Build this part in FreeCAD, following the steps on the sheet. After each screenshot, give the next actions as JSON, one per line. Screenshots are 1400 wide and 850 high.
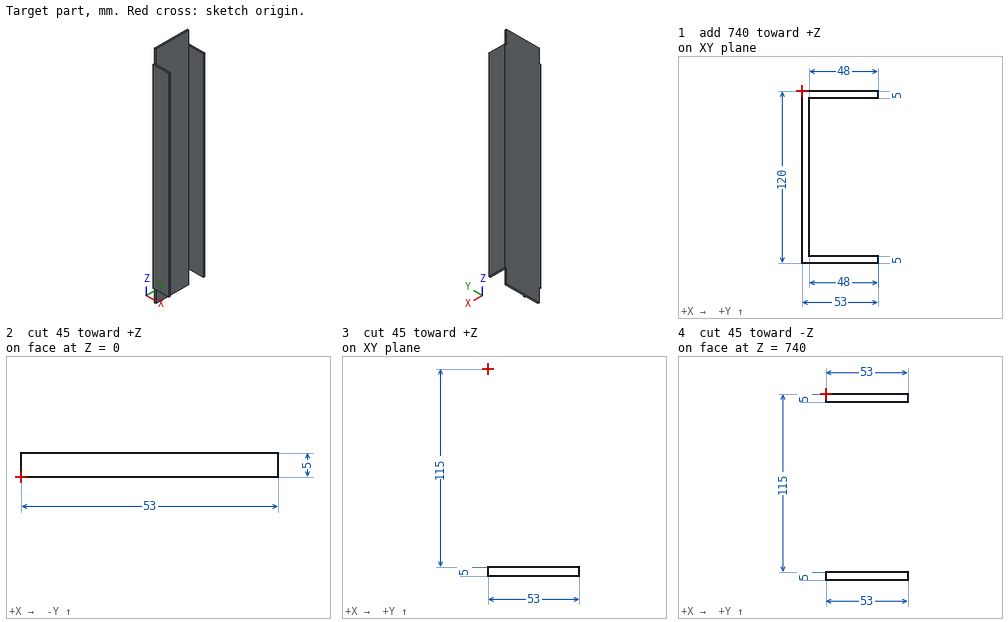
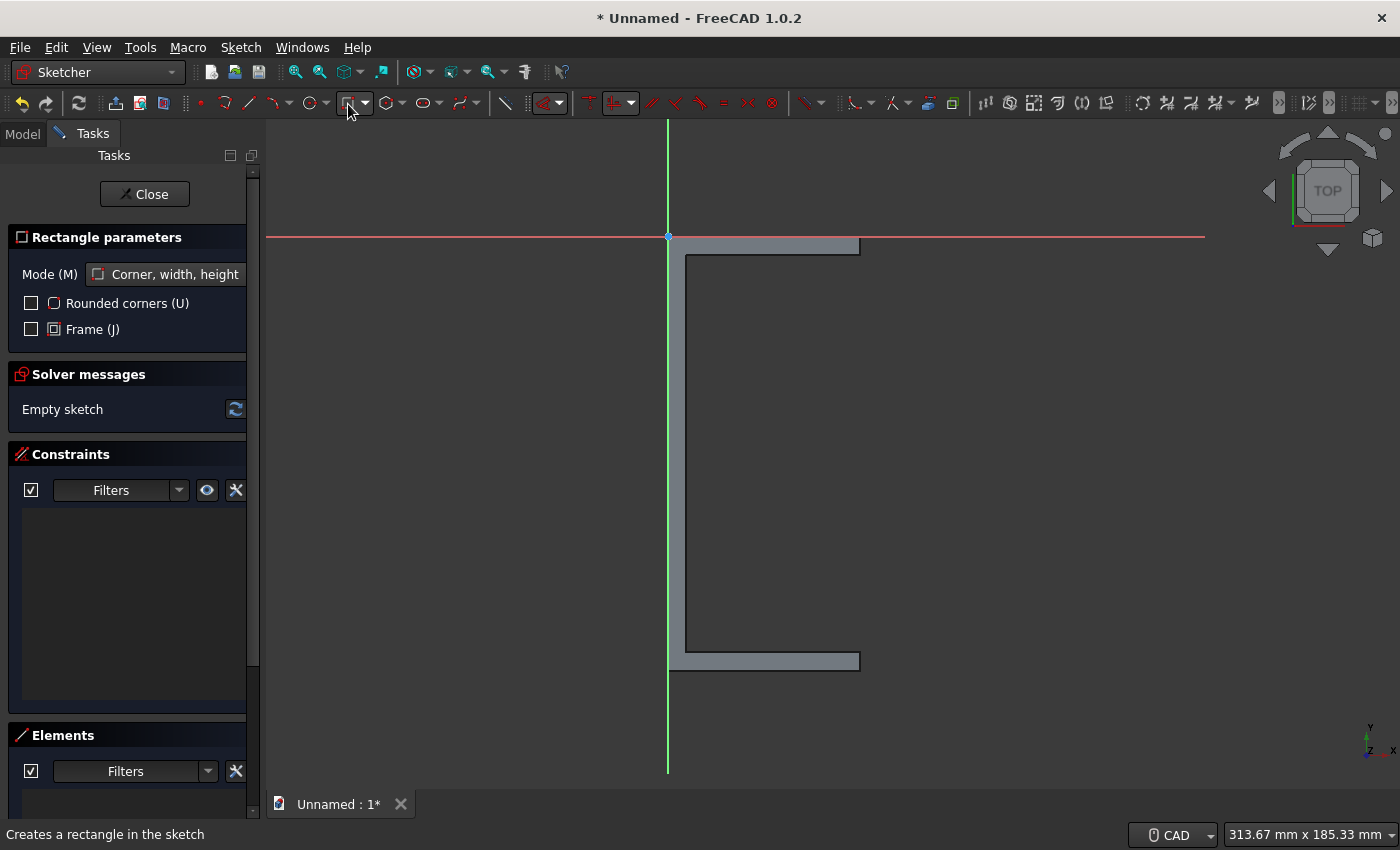
{"action": "left_click", "coordinate": [668, 237]}
{"action": "left_click", "coordinate": [860, 255]}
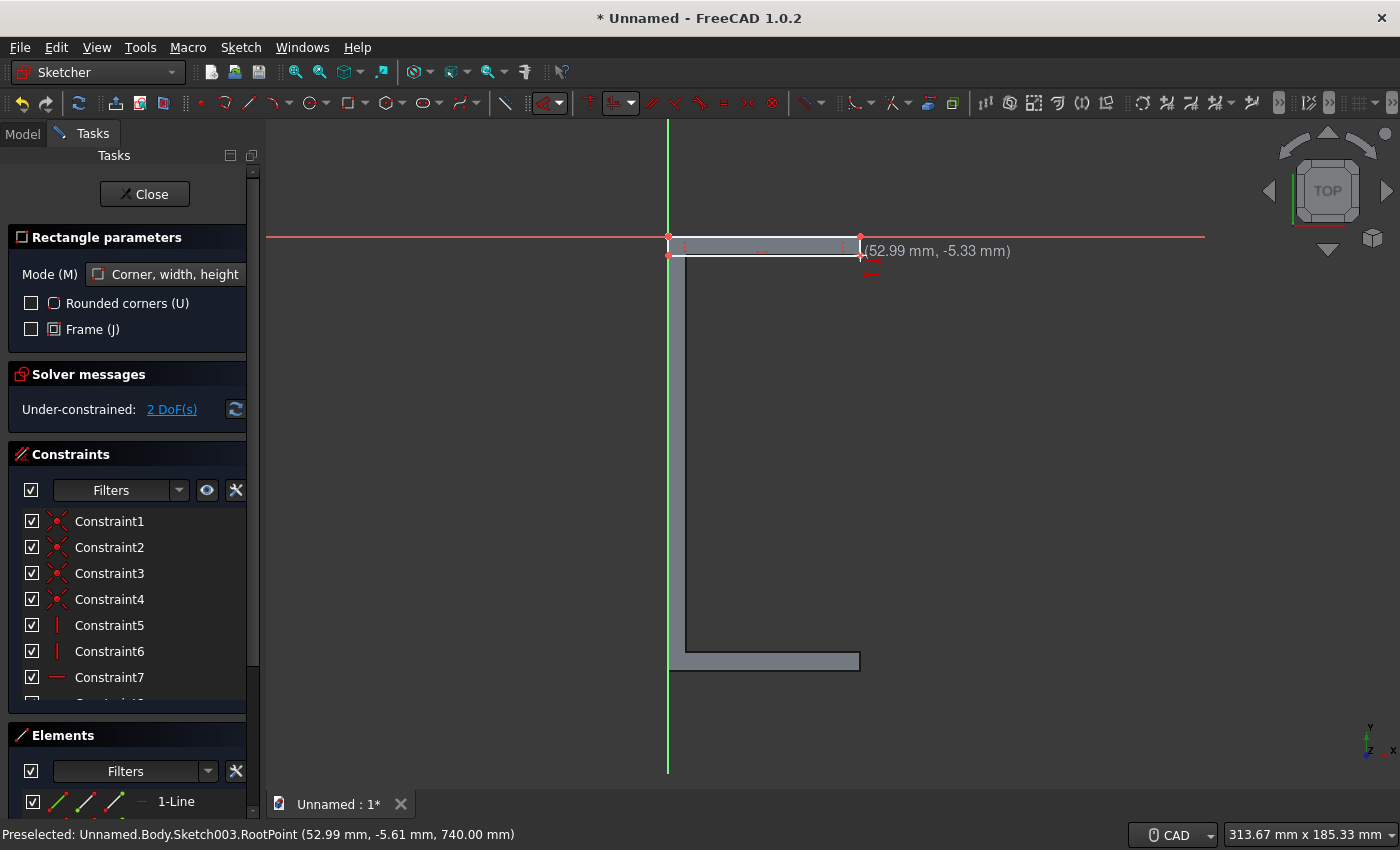
{"action": "left_click", "coordinate": [668, 652]}
{"action": "left_click", "coordinate": [860, 671]}
{"action": "key", "text": "Escape"}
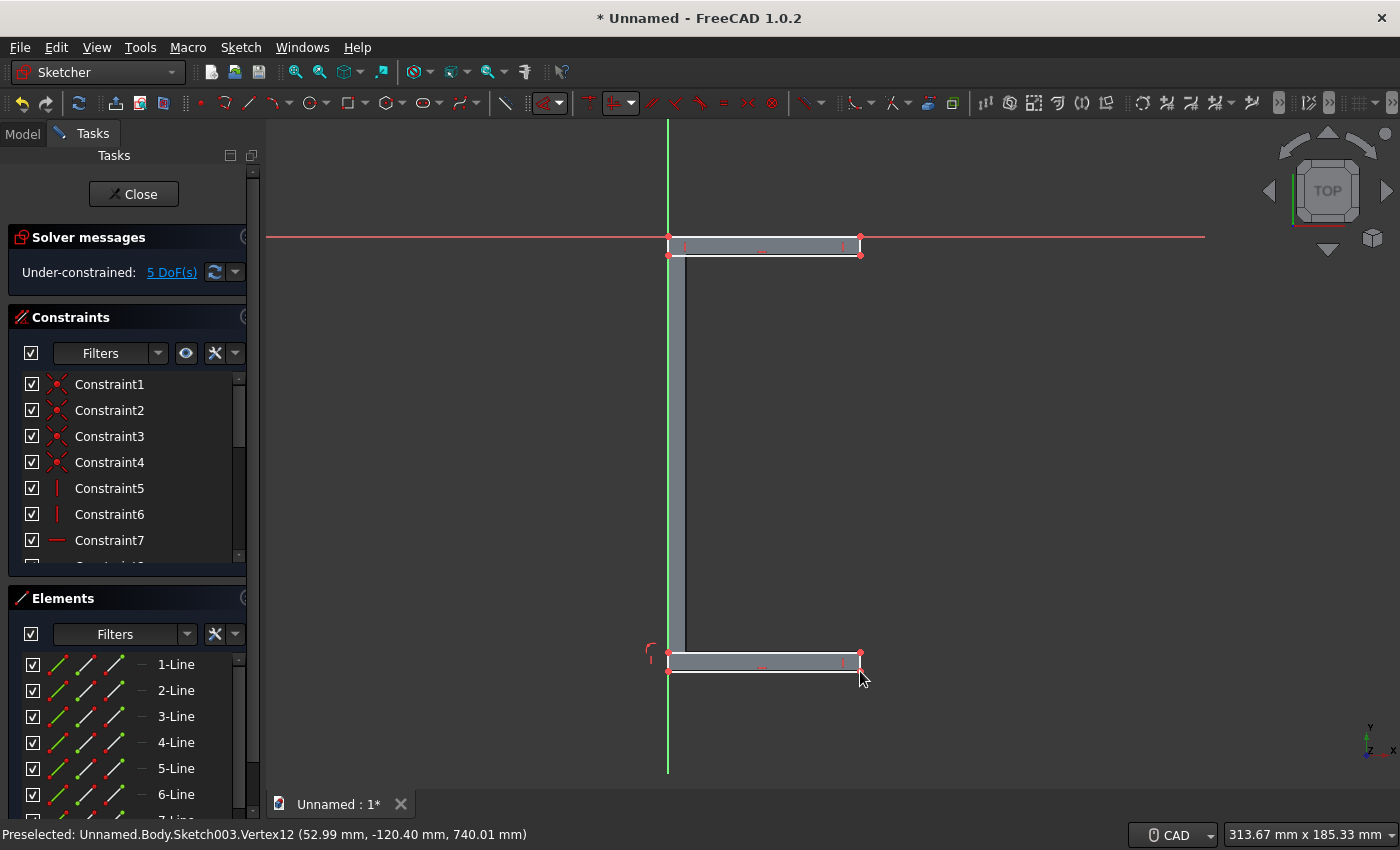
{"action": "scroll", "coordinate": [668, 246], "scroll_direction": "up", "scroll_amount": 4}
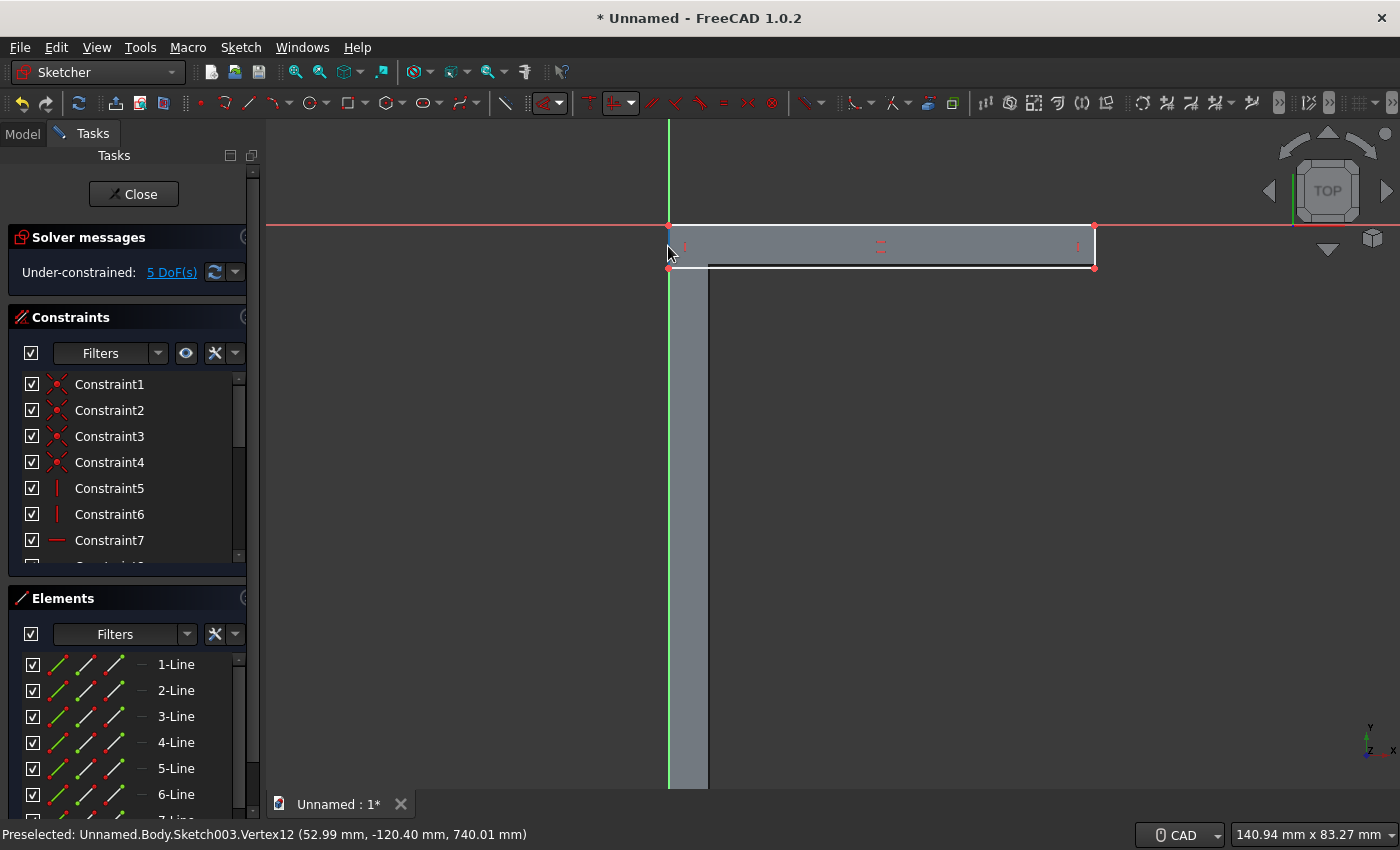
{"action": "left_click", "coordinate": [669, 247]}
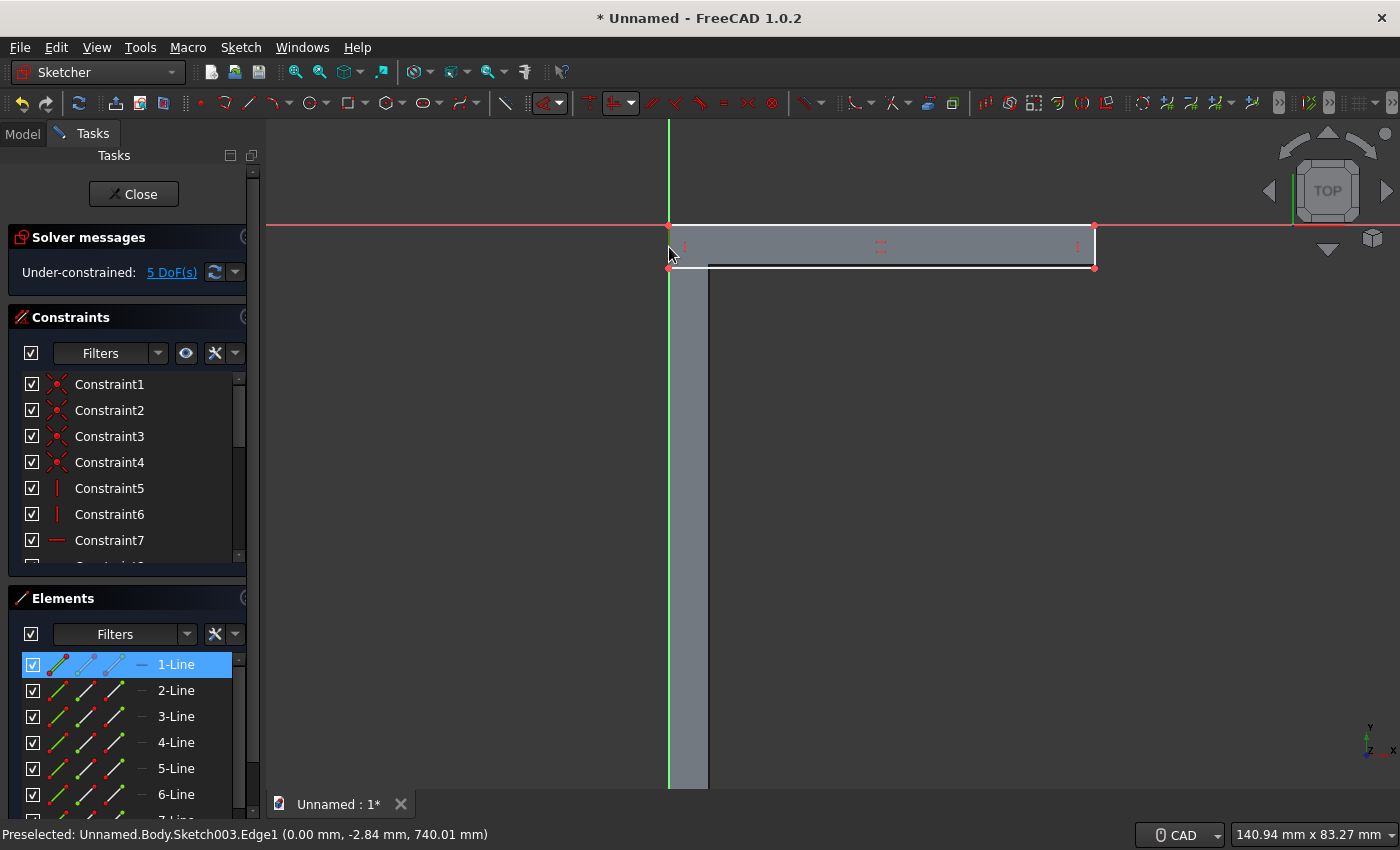
{"action": "left_click", "coordinate": [562, 104]}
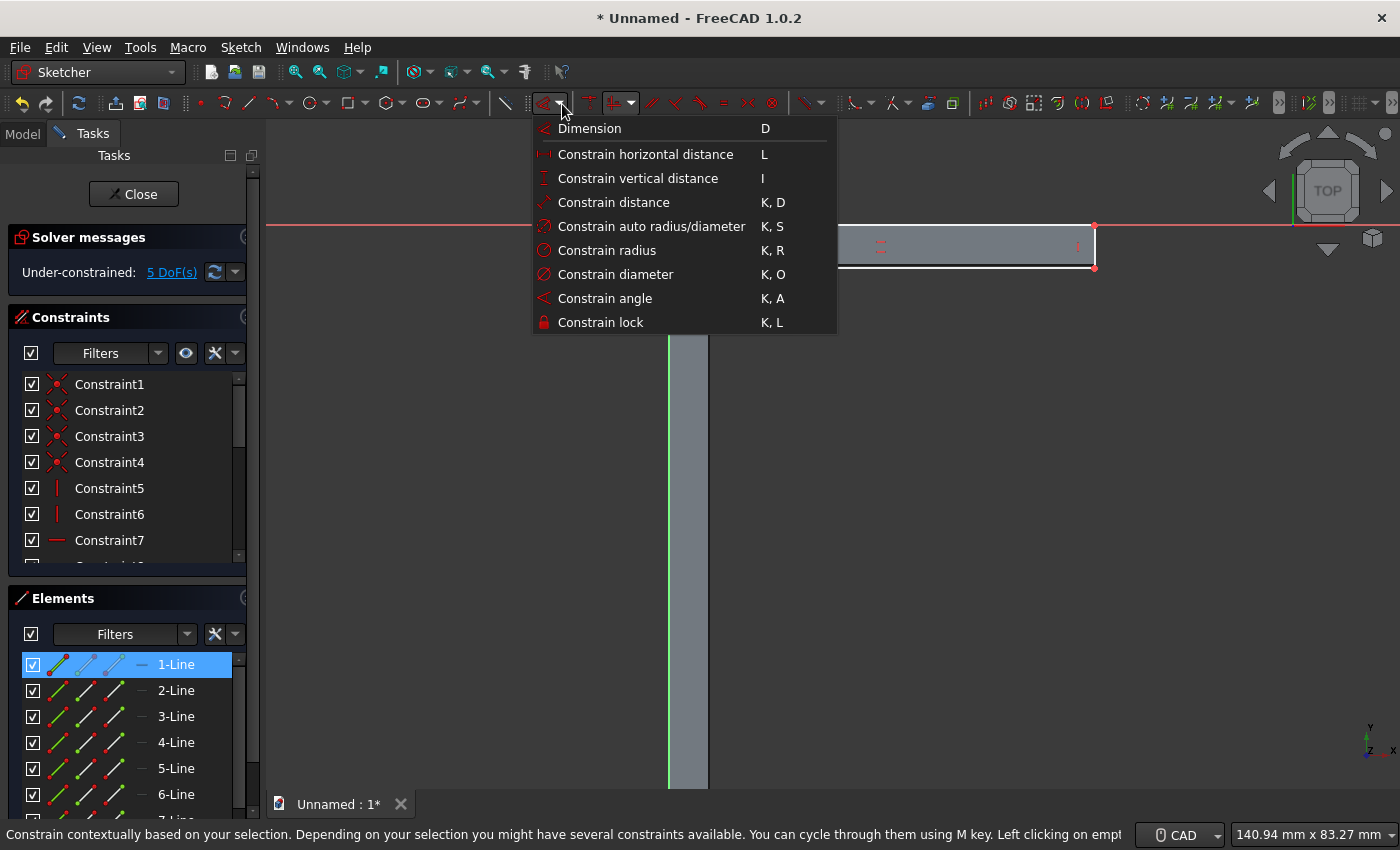
{"action": "left_click", "coordinate": [685, 178]}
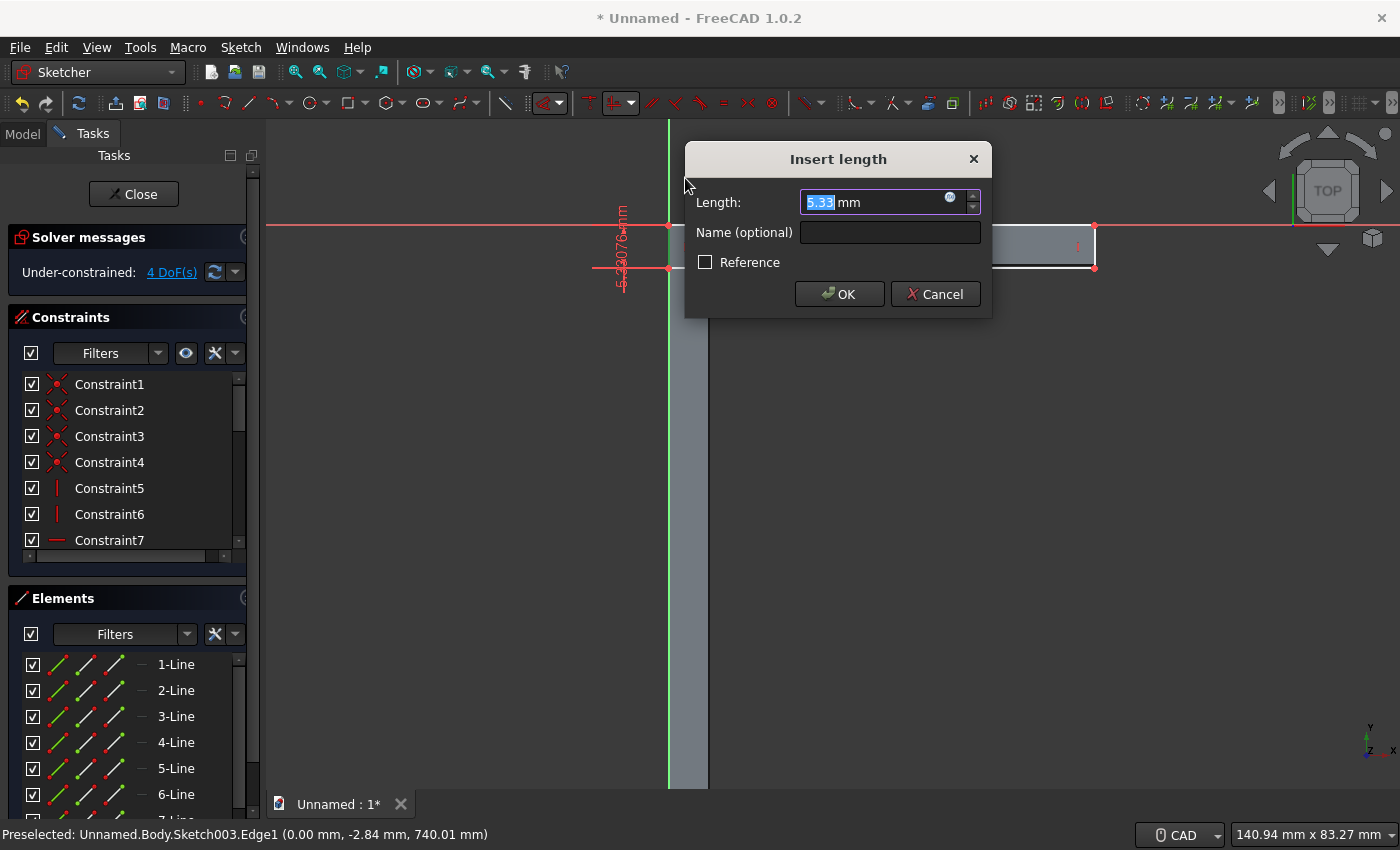
{"action": "type", "text": "5"}
{"action": "key", "text": "Return"}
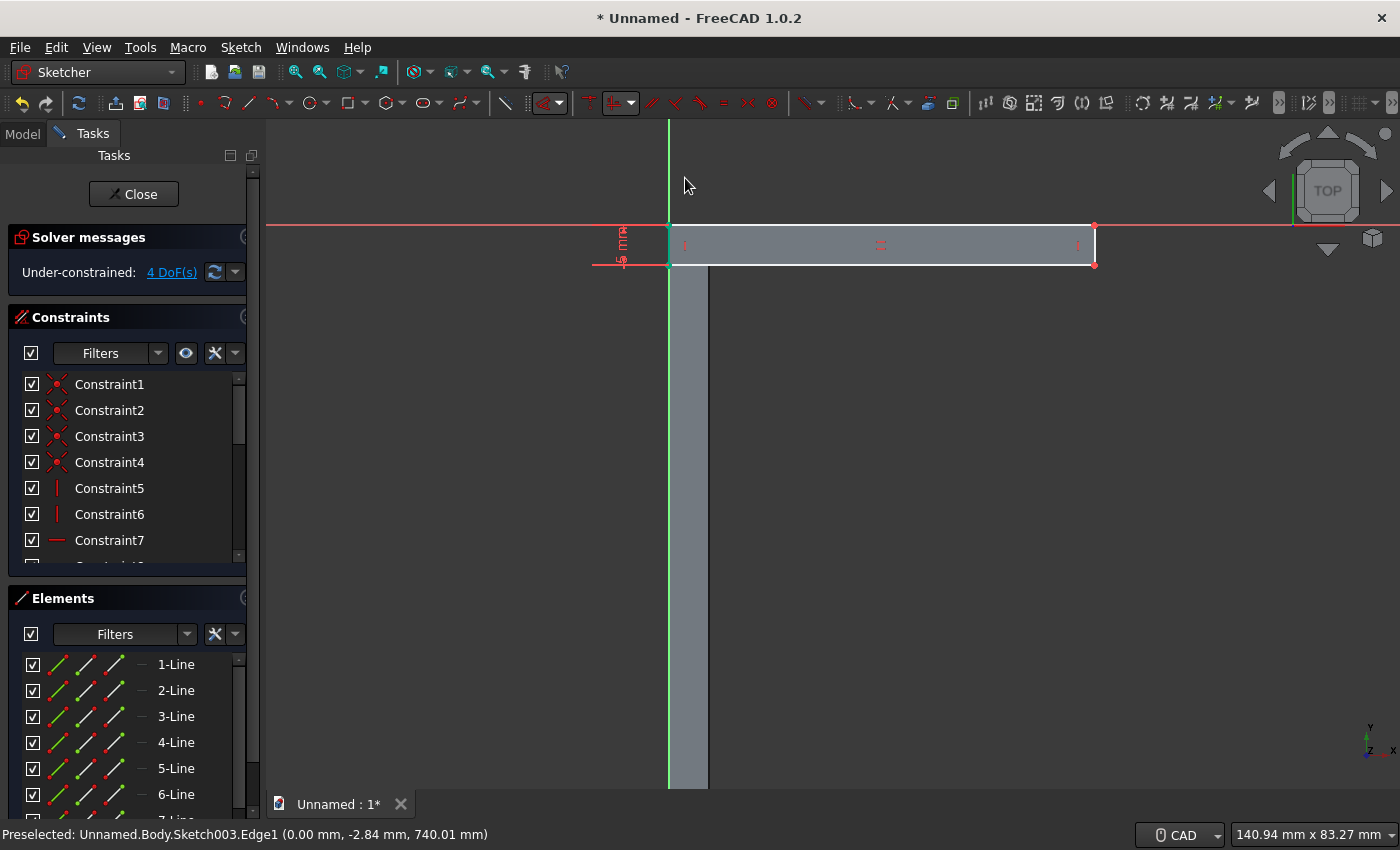
{"action": "scroll", "coordinate": [669, 247], "scroll_direction": "down", "scroll_amount": 4}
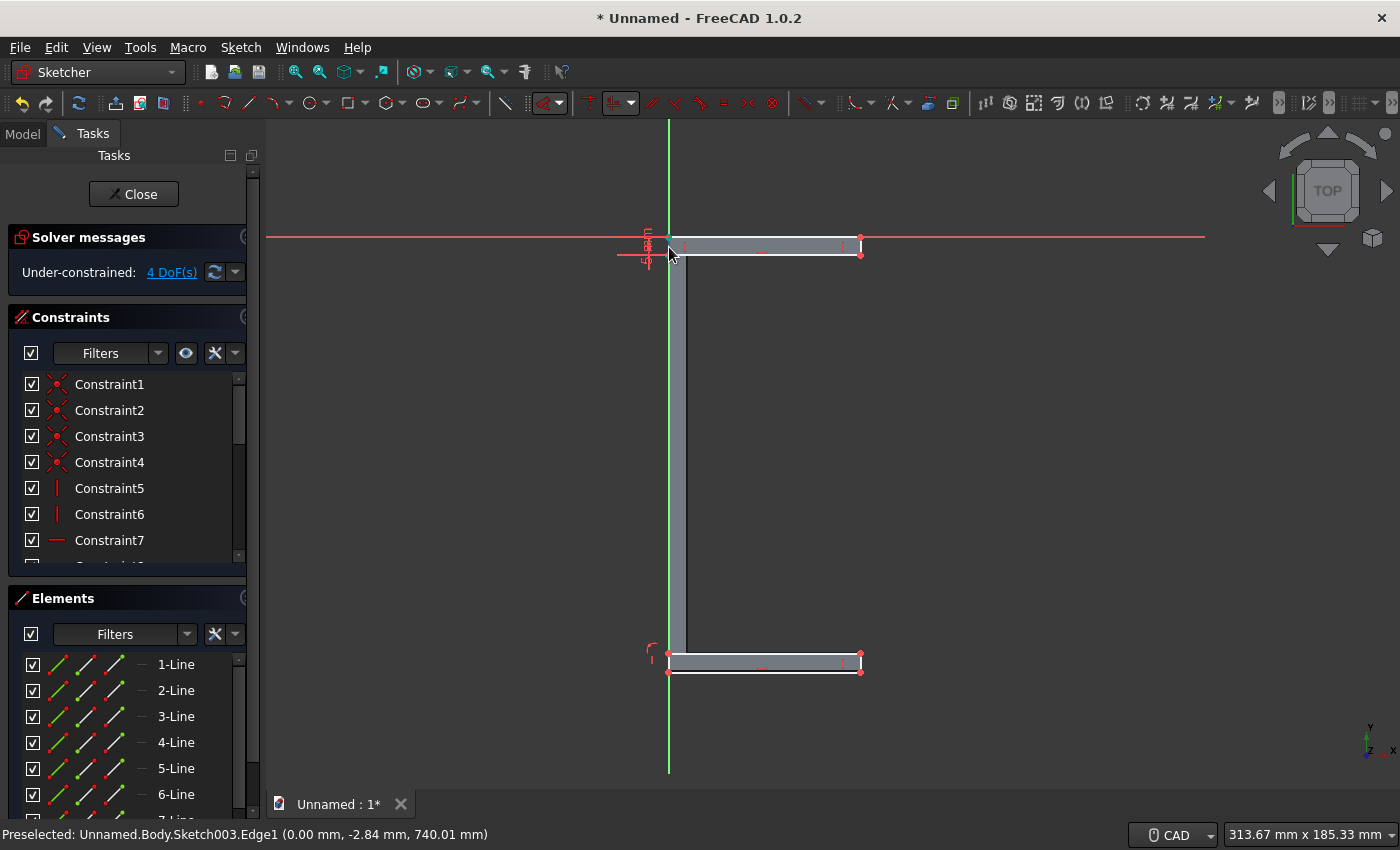
{"action": "scroll", "coordinate": [669, 659], "scroll_direction": "up", "scroll_amount": 5}